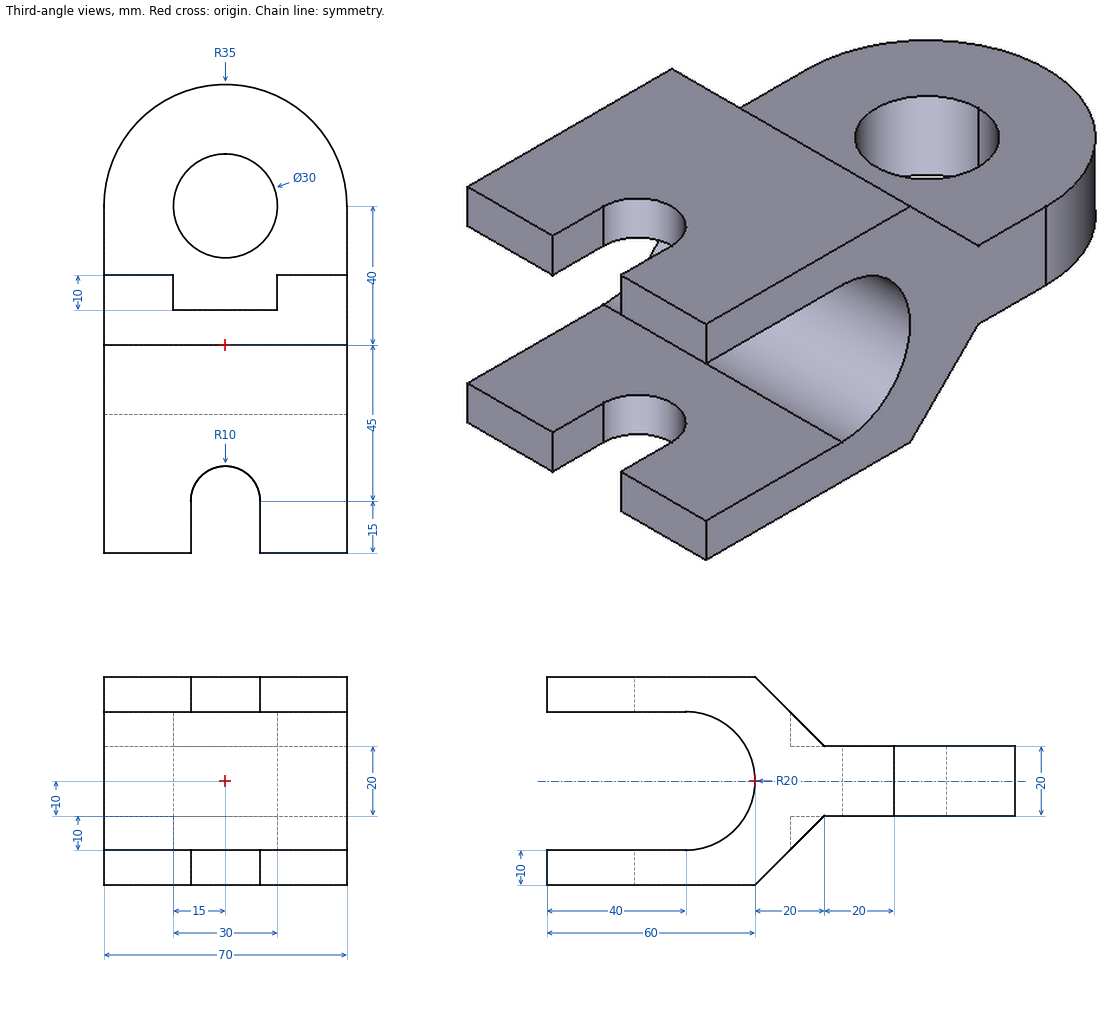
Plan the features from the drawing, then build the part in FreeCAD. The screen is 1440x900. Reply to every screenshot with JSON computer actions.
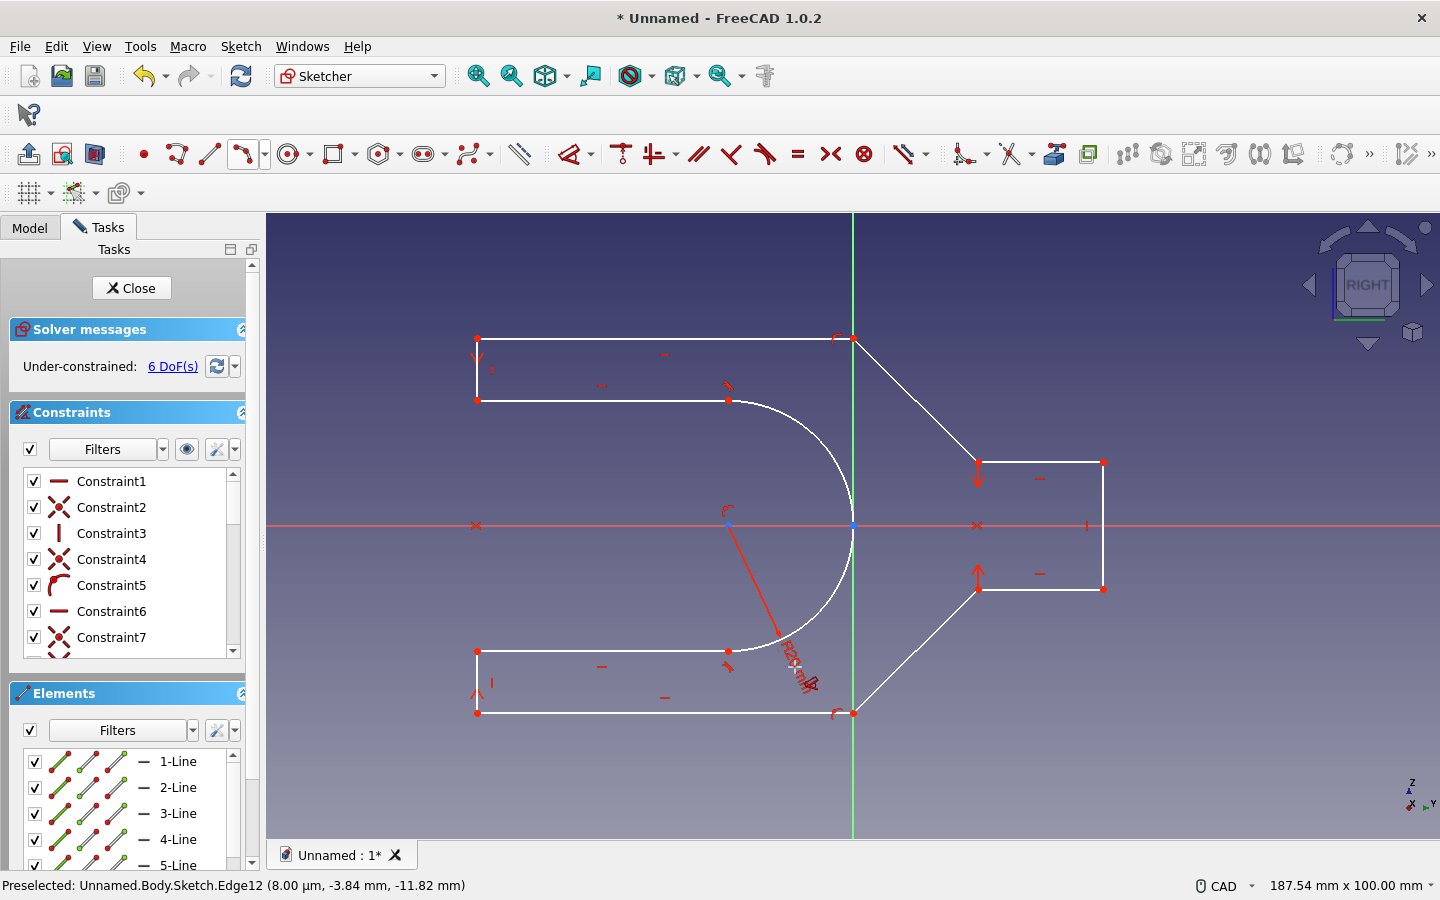
{"action": "left_click", "coordinate": [653, 651]}
{"action": "left_click", "coordinate": [603, 685]}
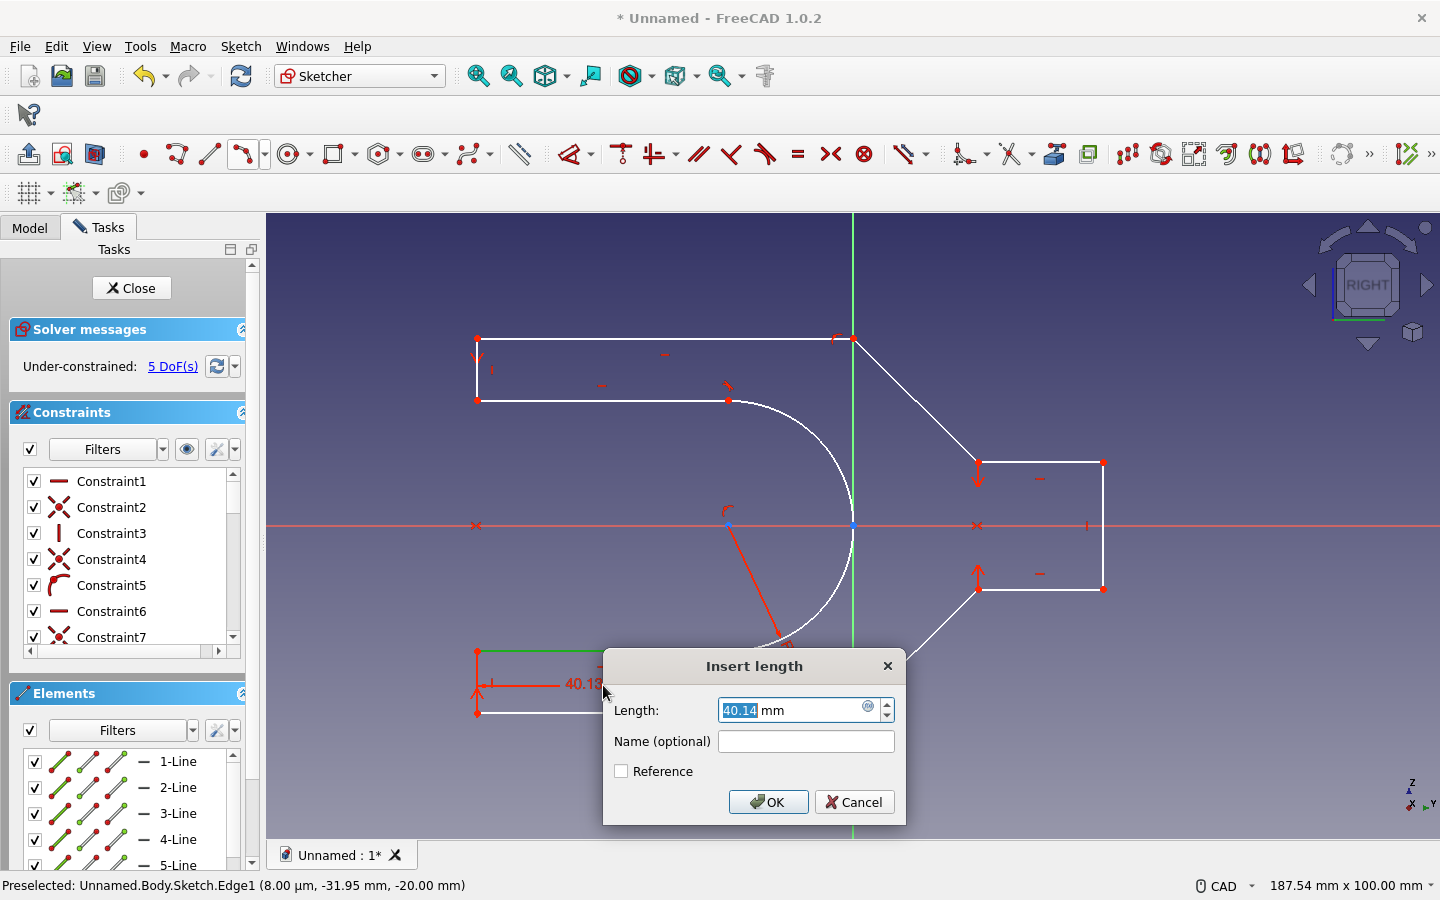
{"action": "type", "text": "40"}
{"action": "key", "text": "Return"}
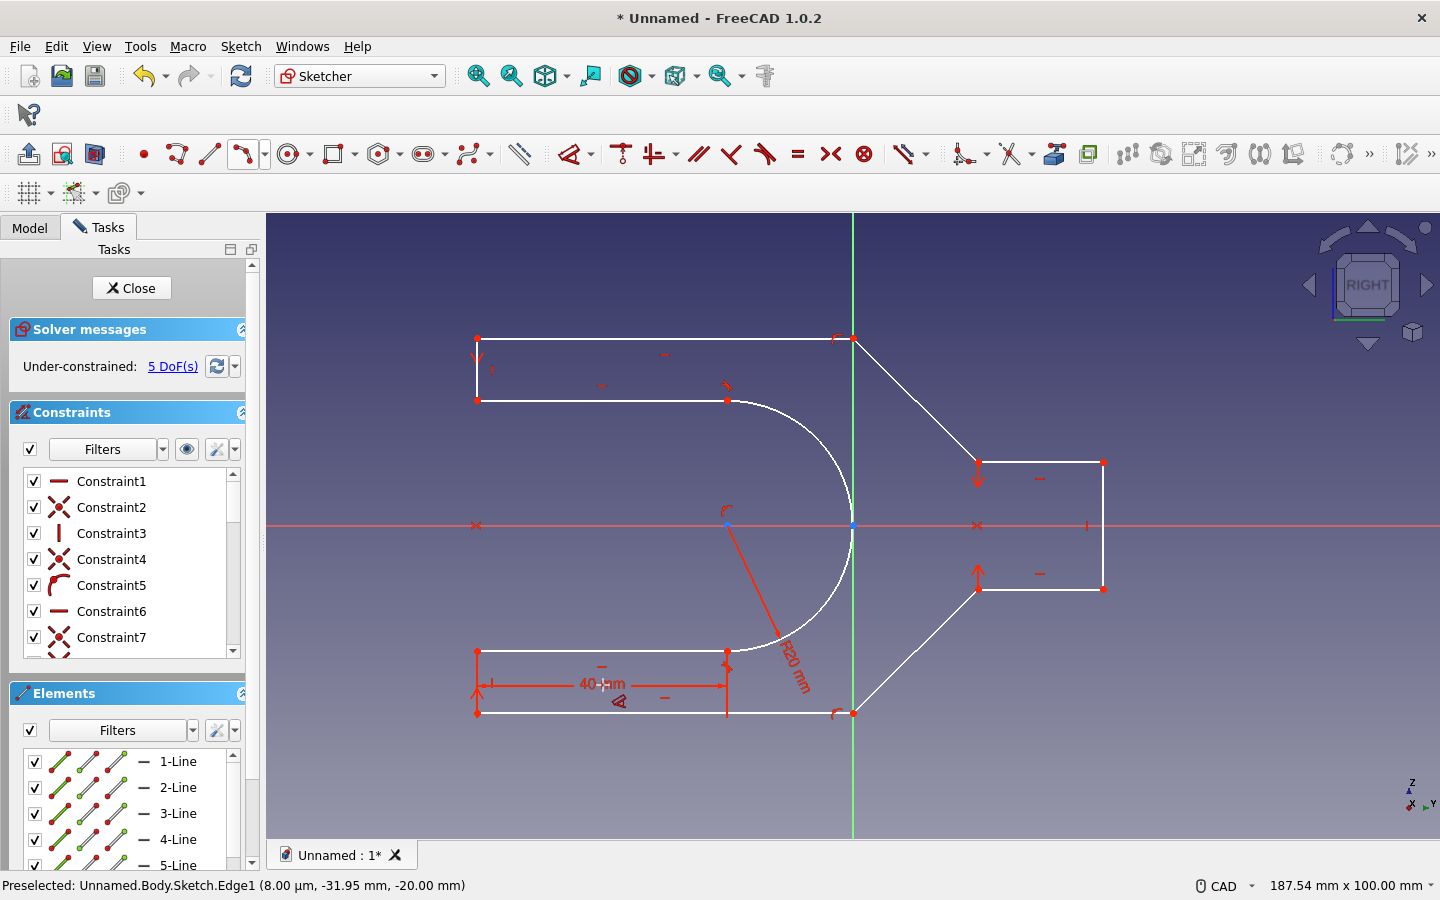
{"action": "left_click", "coordinate": [477, 670]}
{"action": "left_click", "coordinate": [443, 682]}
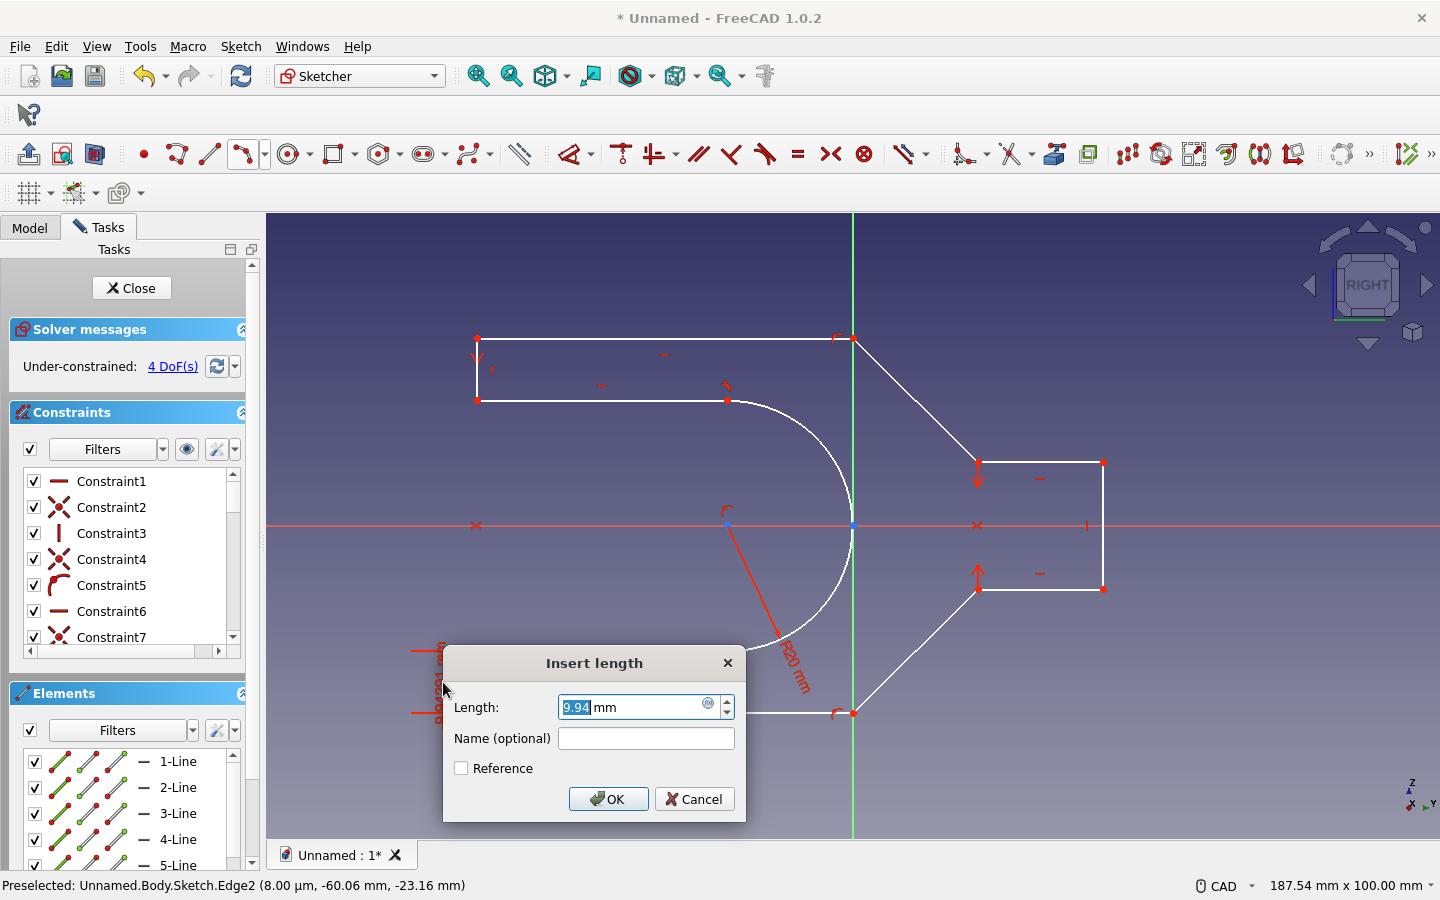
{"action": "type", "text": "10"}
{"action": "key", "text": "Return"}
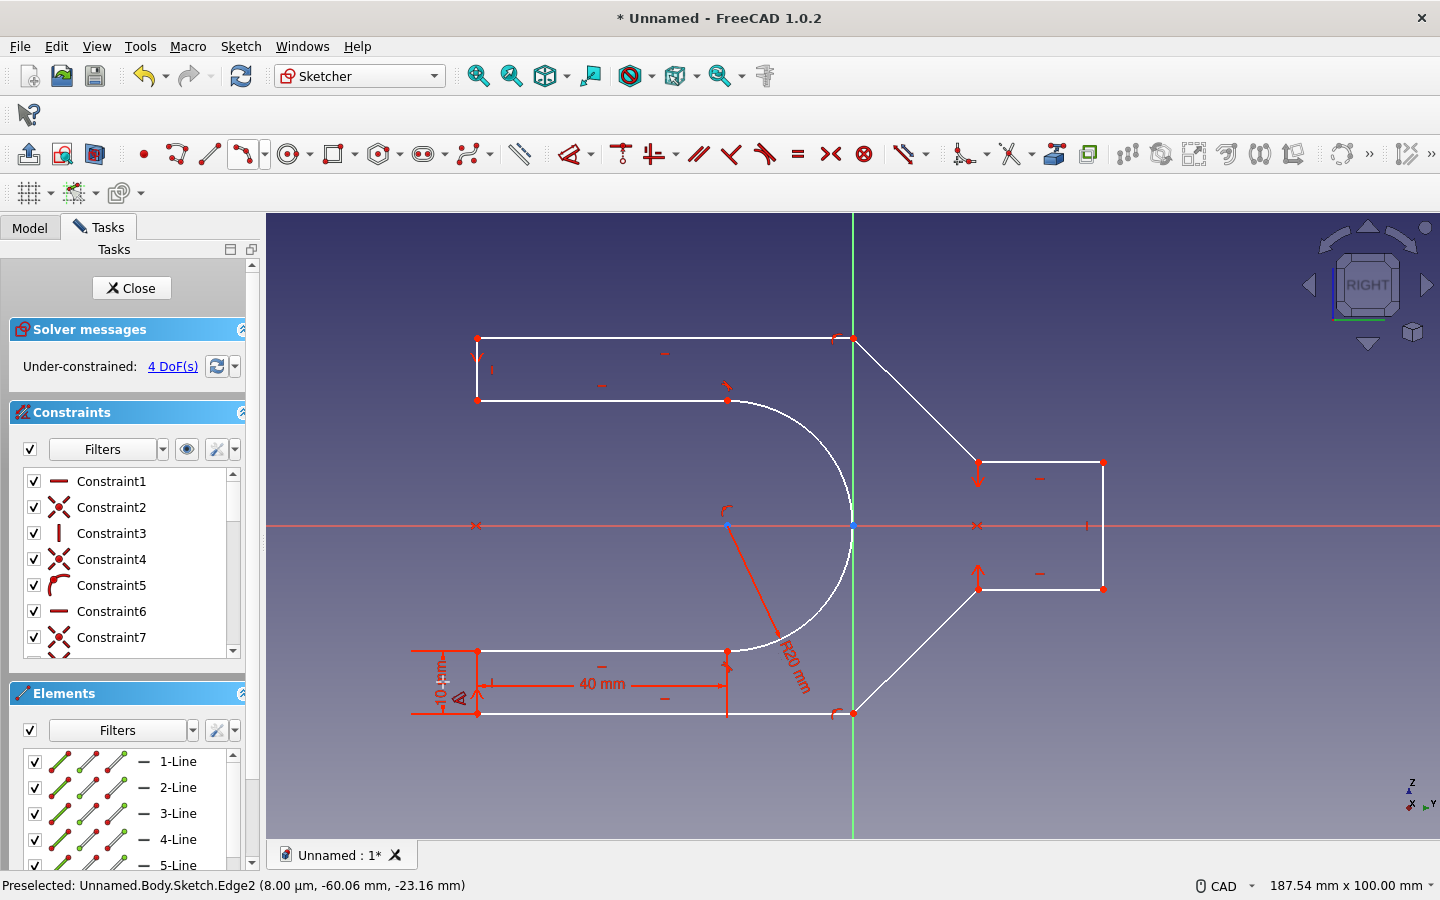
{"action": "left_click", "coordinate": [590, 714]}
{"action": "left_click", "coordinate": [665, 748]}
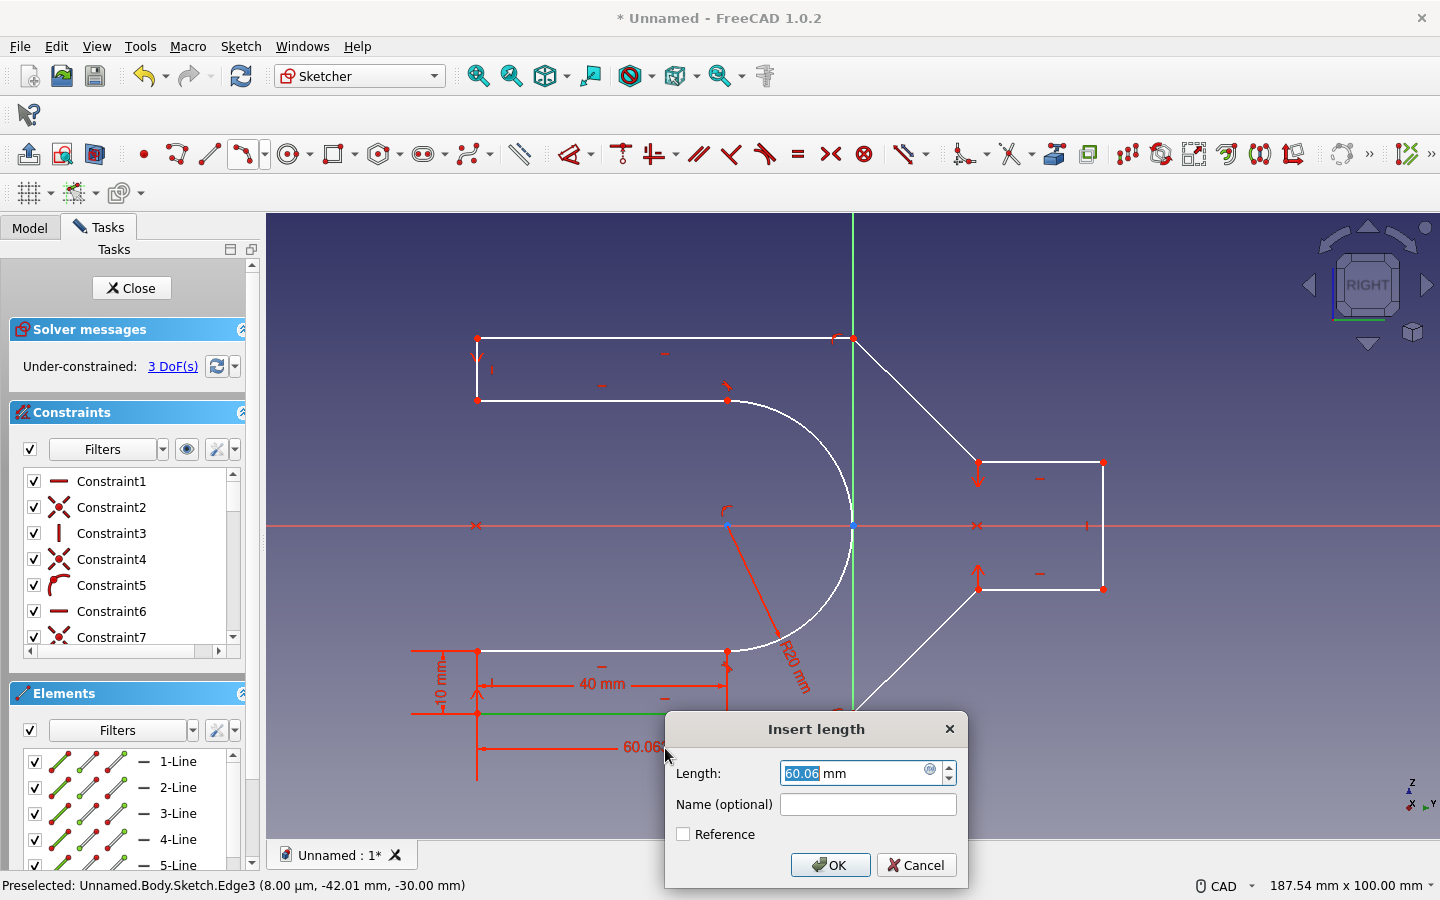
{"action": "type", "text": "60"}
{"action": "key", "text": "Return"}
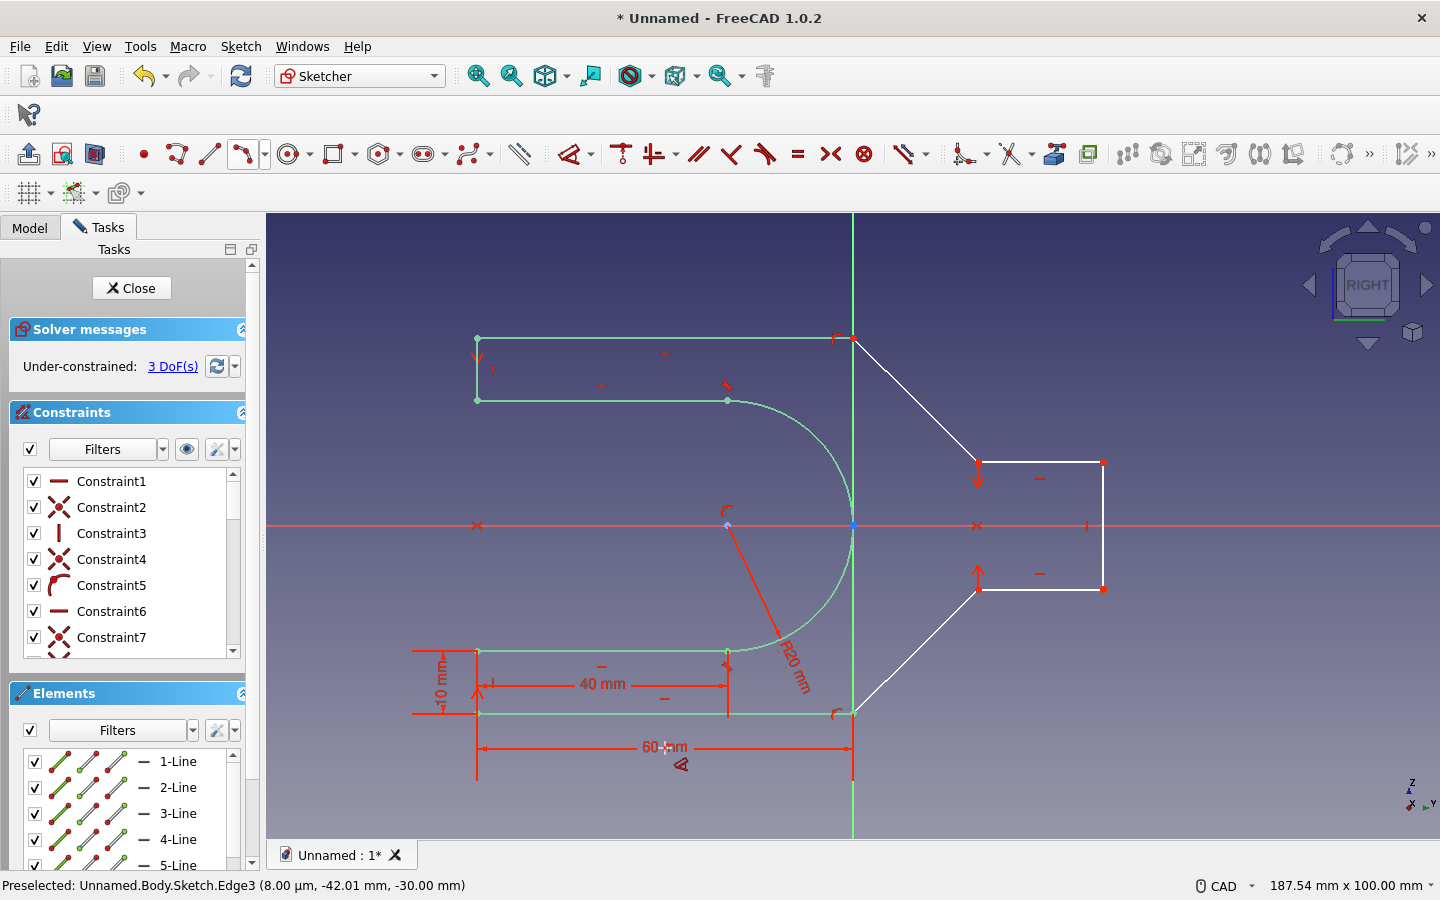
{"action": "left_click", "coordinate": [1015, 590]}
{"action": "left_click", "coordinate": [1040, 624]}